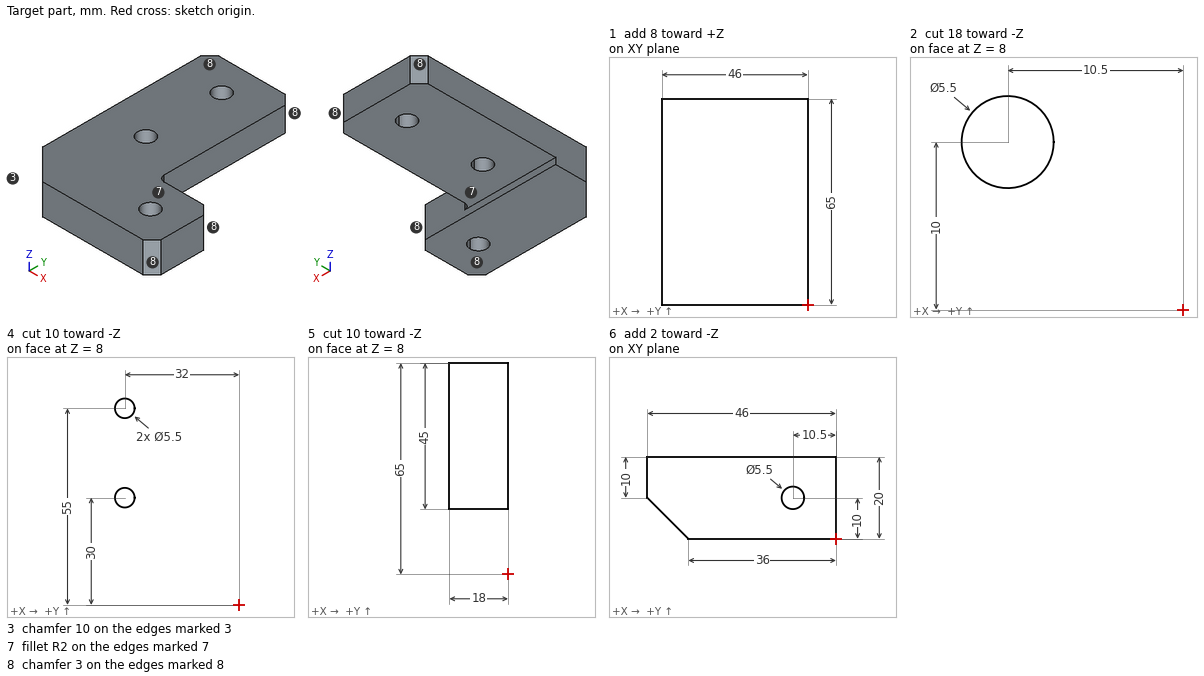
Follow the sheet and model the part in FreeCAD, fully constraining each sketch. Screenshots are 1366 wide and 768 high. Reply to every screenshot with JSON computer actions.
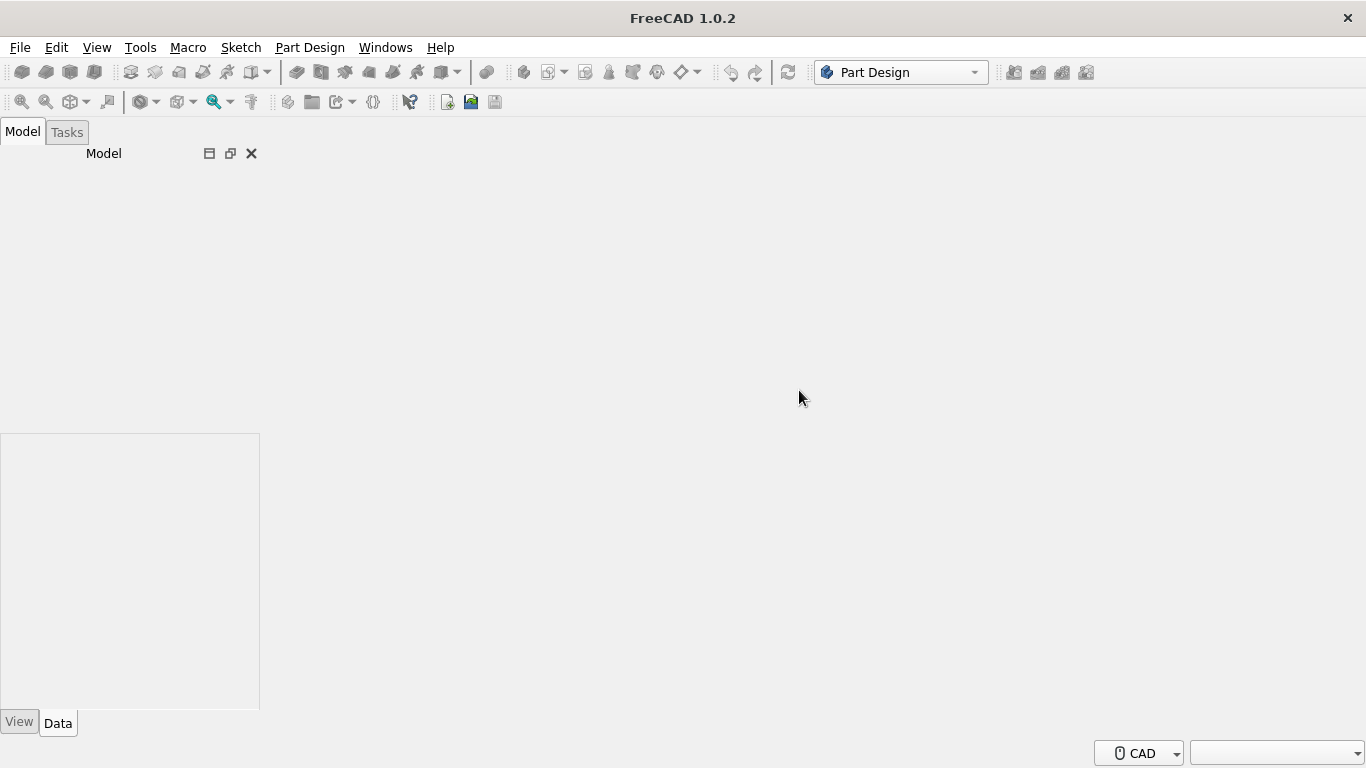
{"action": "left_click", "coordinate": [448, 102]}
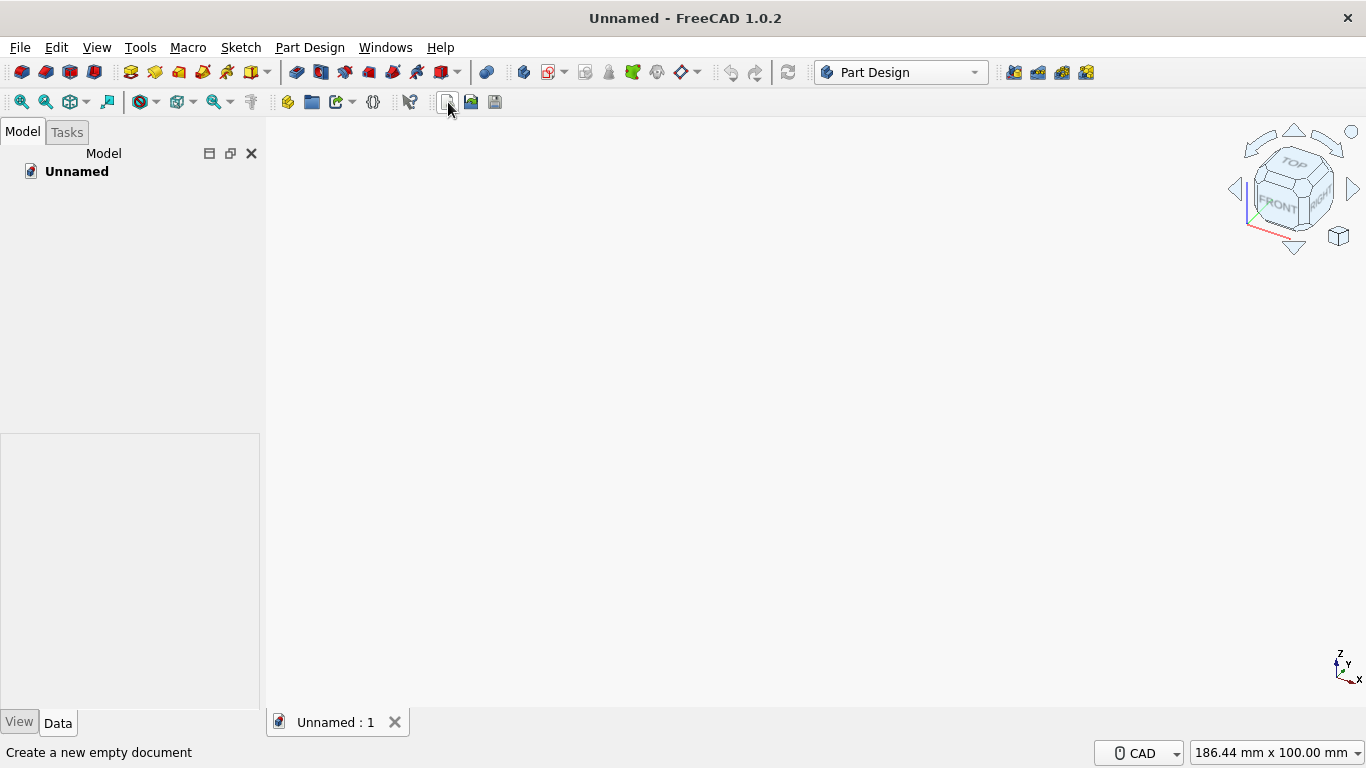
{"action": "left_click", "coordinate": [548, 72]}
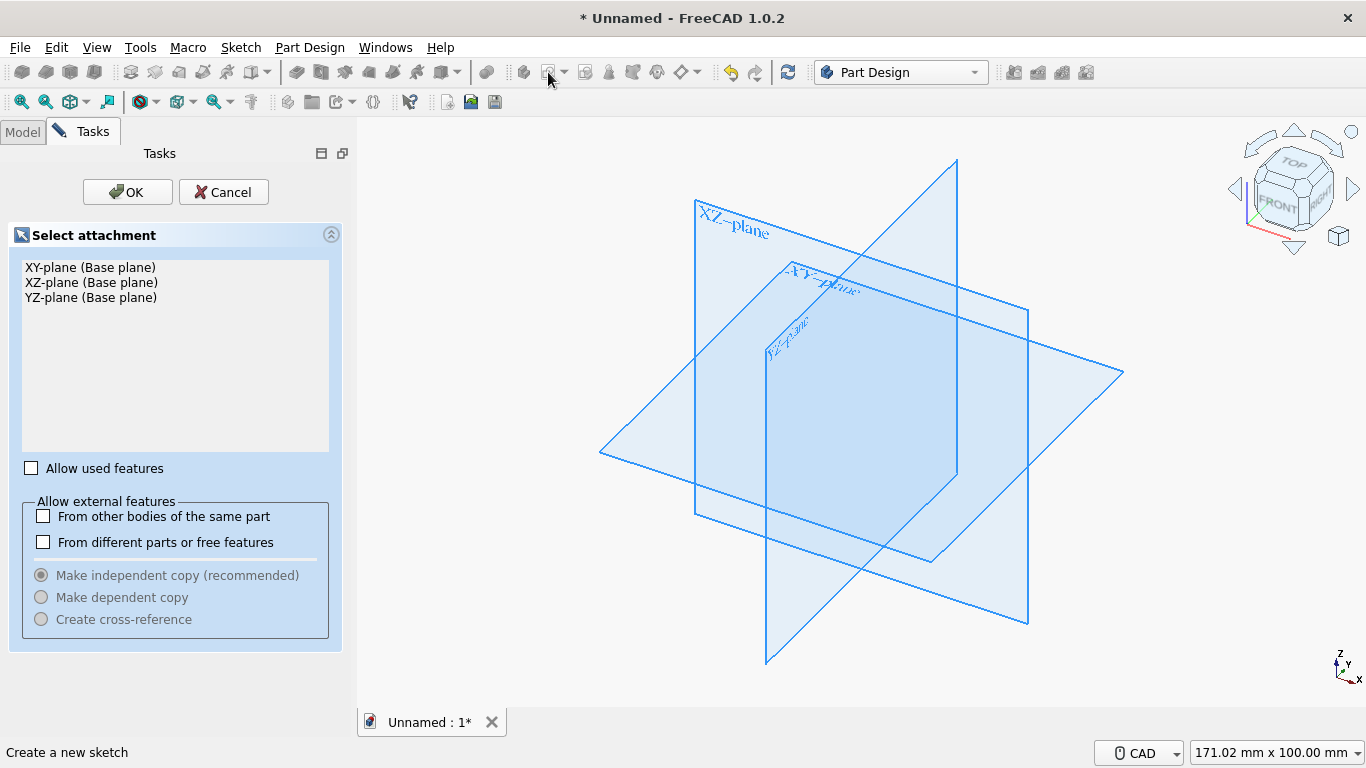
{"action": "left_click", "coordinate": [82, 268]}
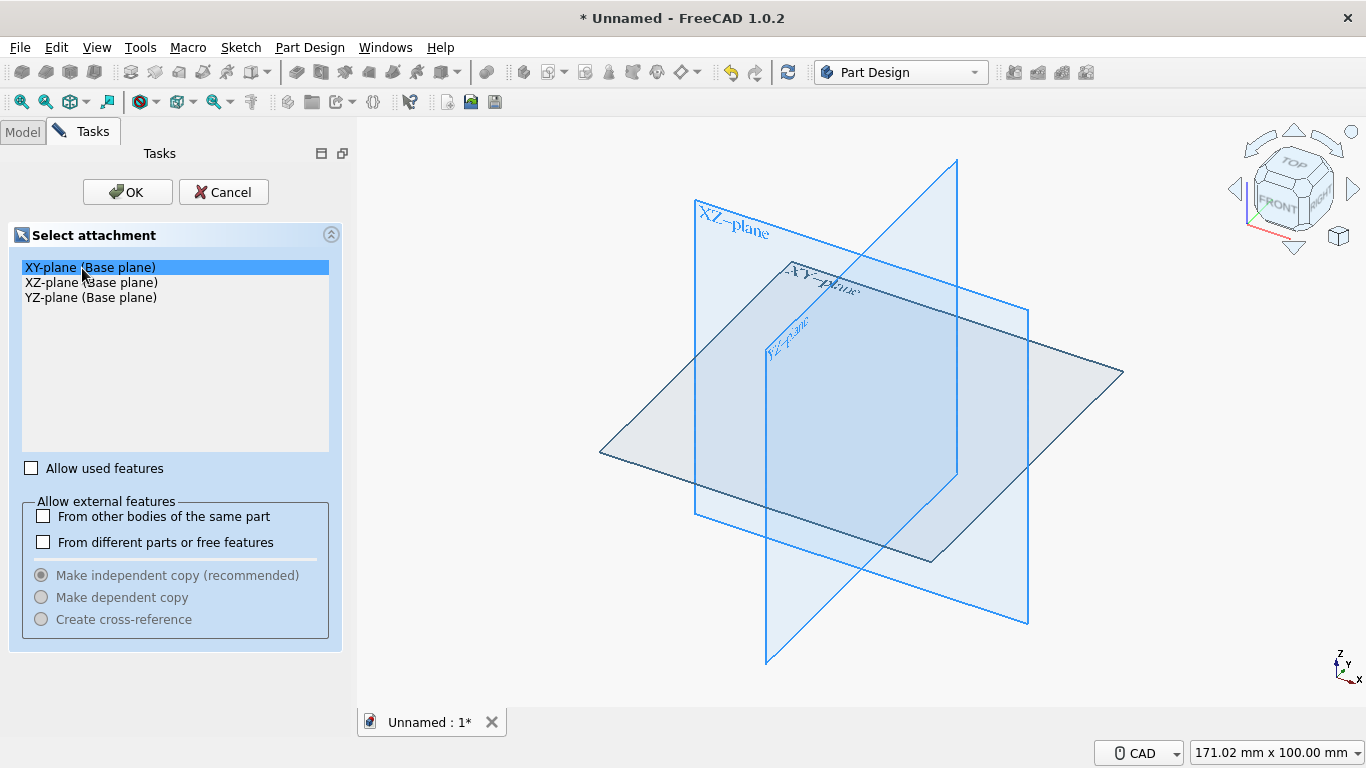
{"action": "left_click", "coordinate": [128, 192]}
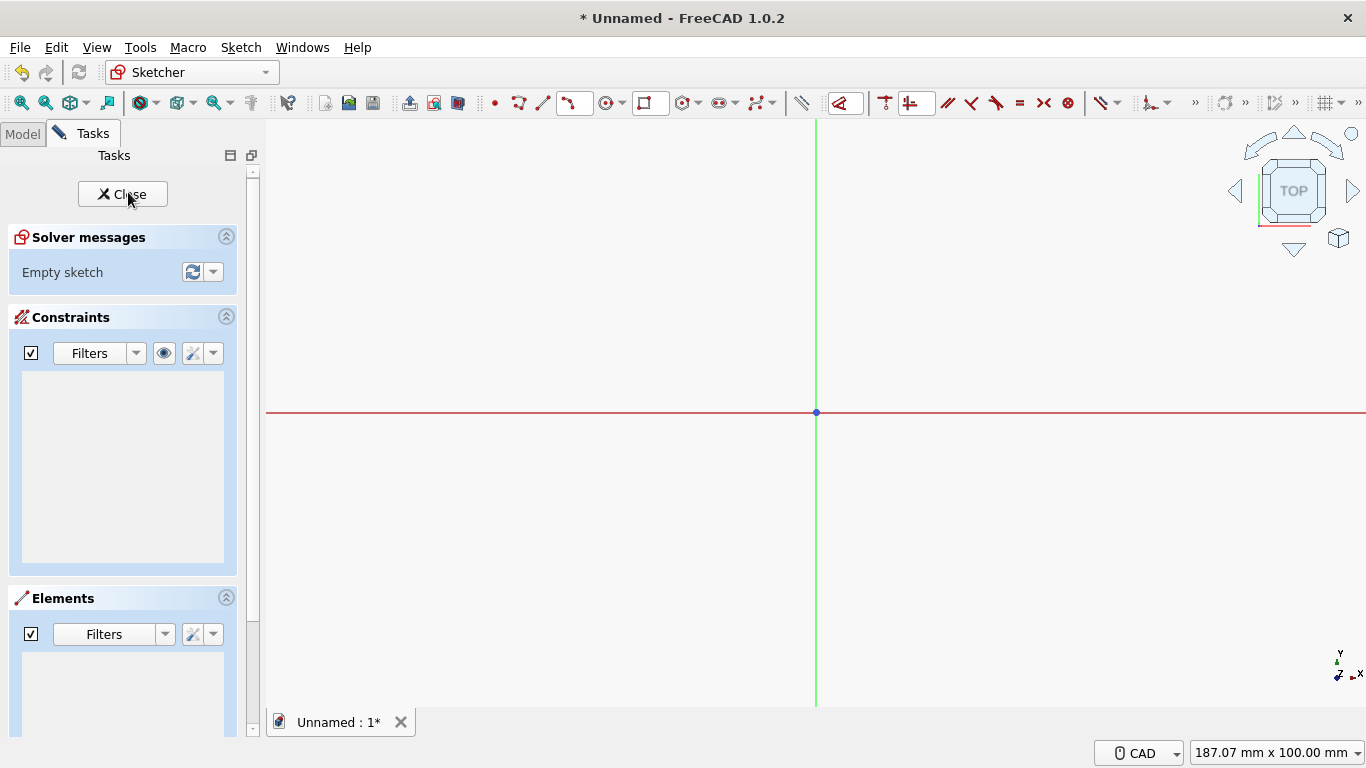
{"action": "scroll", "coordinate": [883, 679], "scroll_direction": "down", "scroll_amount": 2}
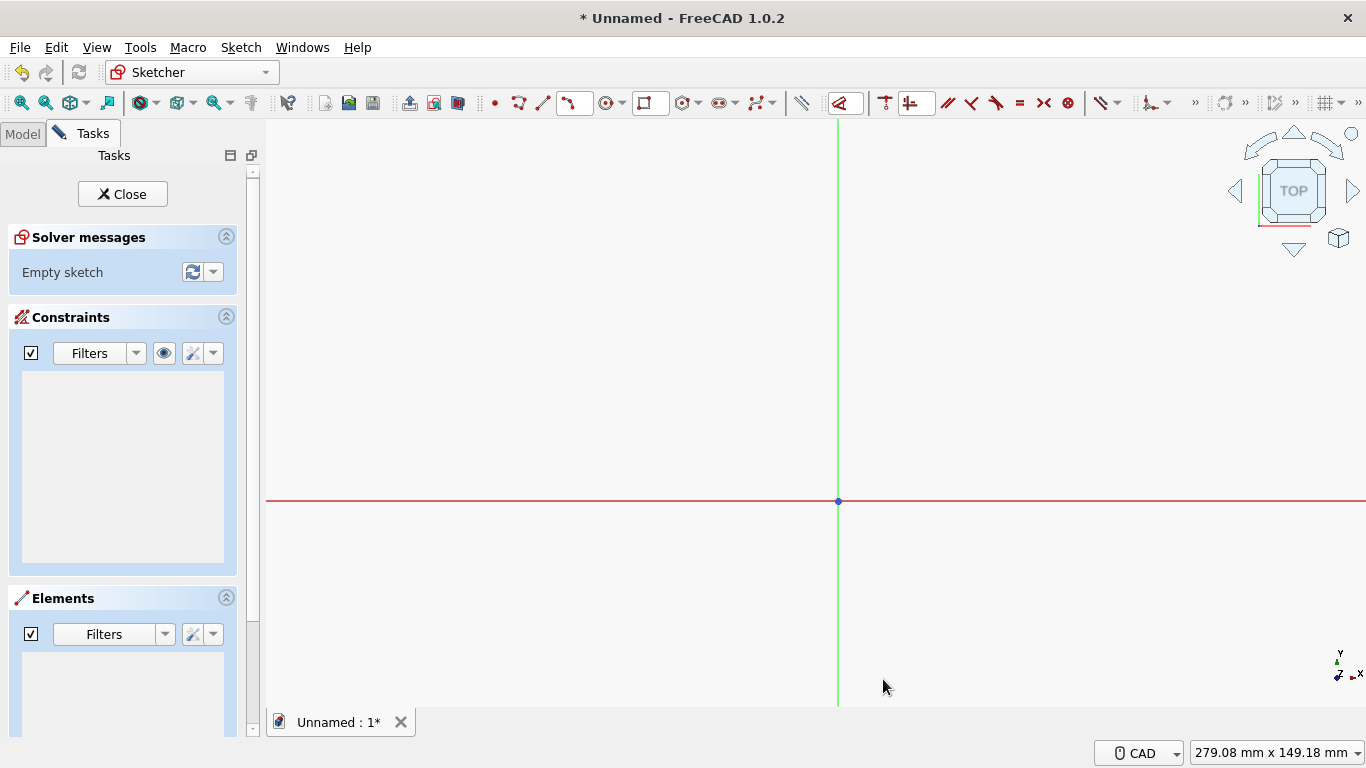
{"action": "scroll", "coordinate": [748, 291], "scroll_direction": "up", "scroll_amount": 2}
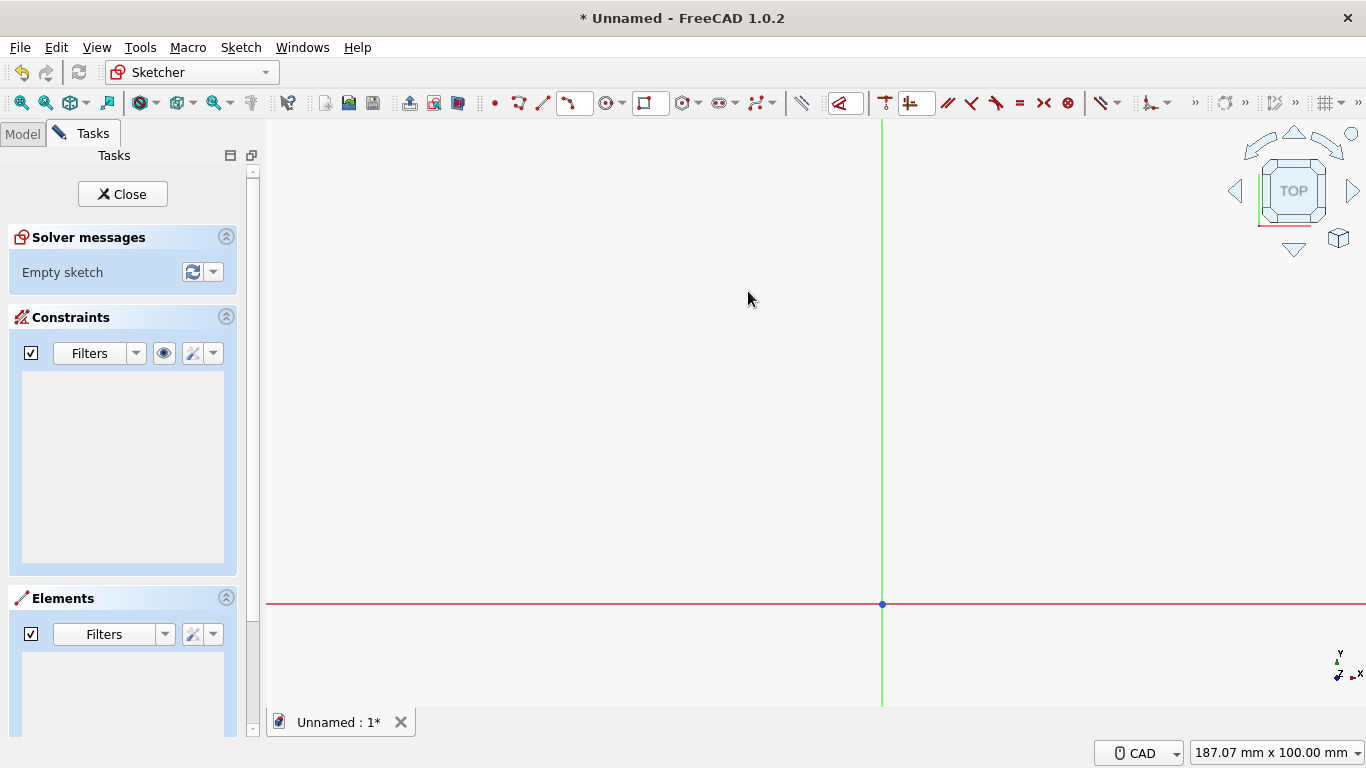
{"action": "key", "text": "g r"}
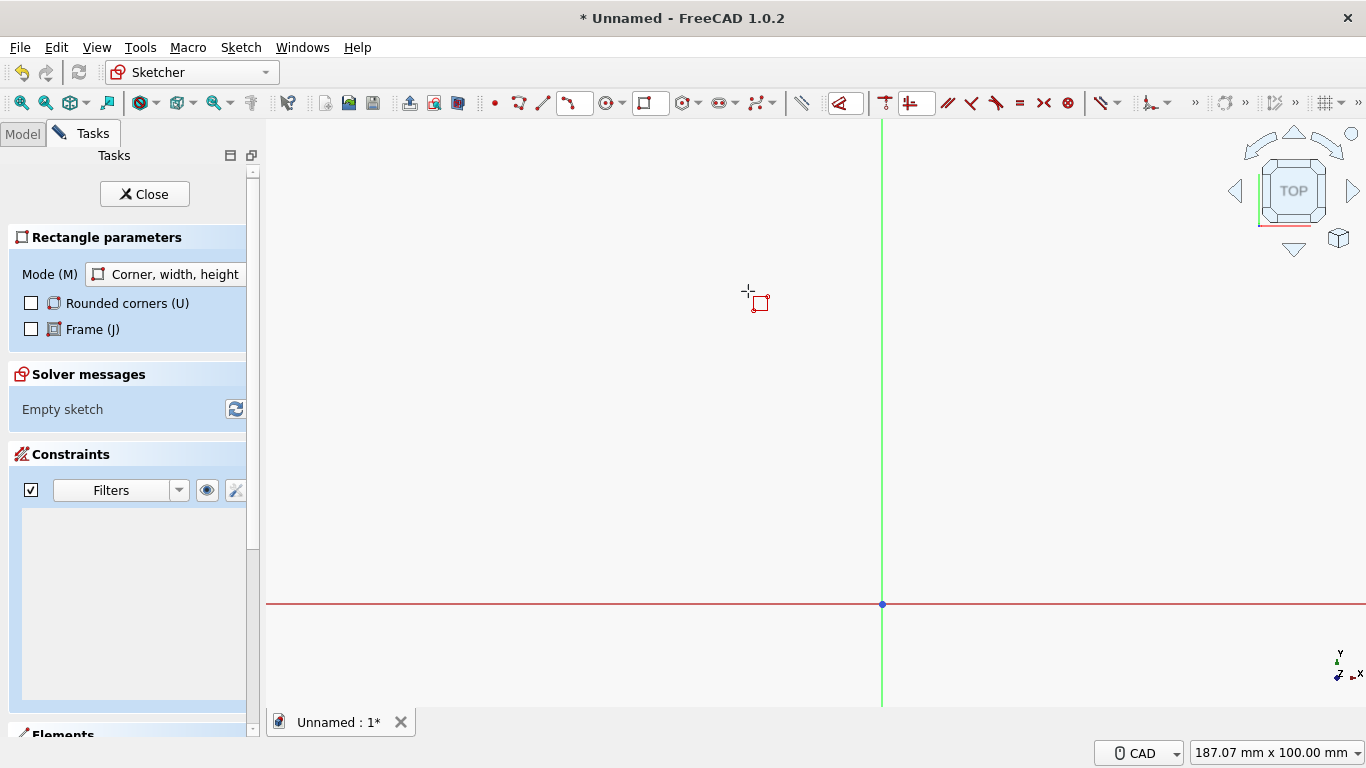
{"action": "left_click", "coordinate": [882, 604]}
{"action": "left_click", "coordinate": [612, 222]}
{"action": "key", "text": "Escape"}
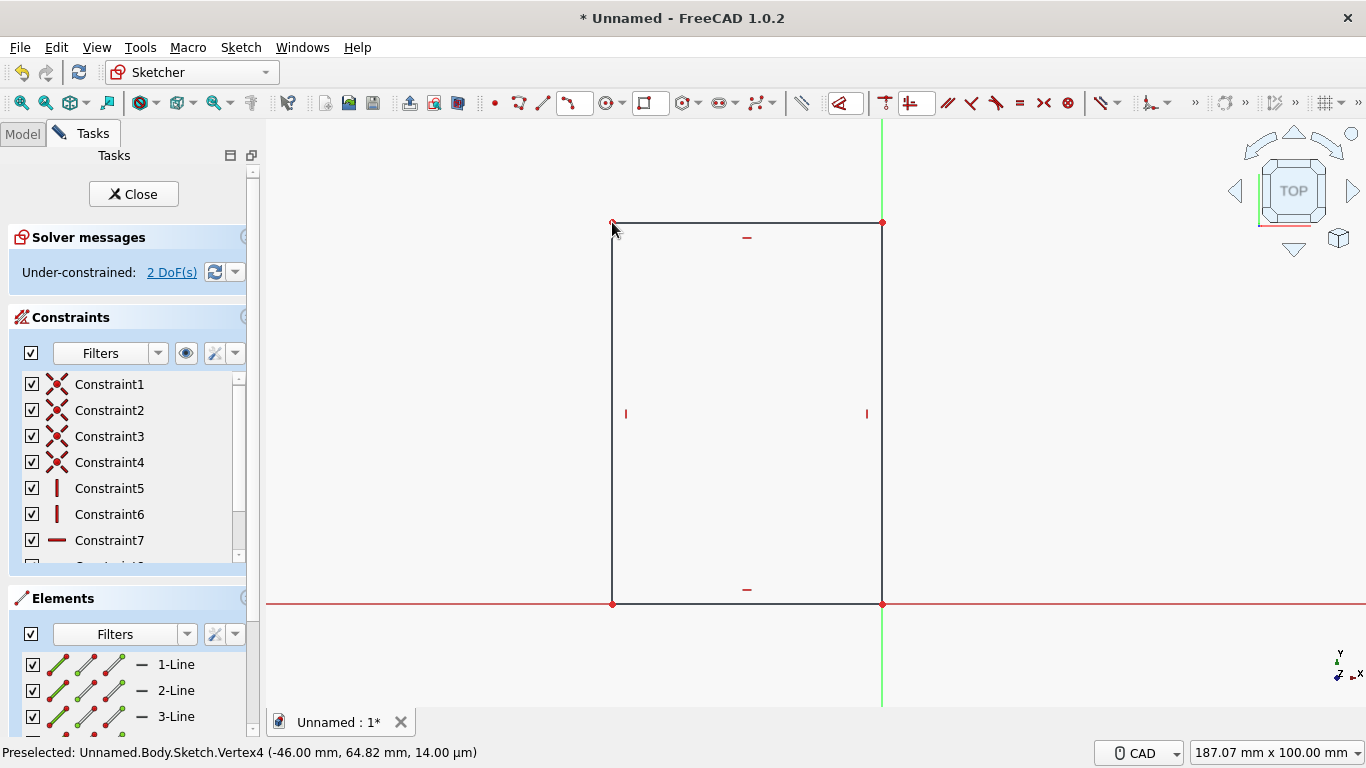
{"action": "left_click", "coordinate": [882, 490]}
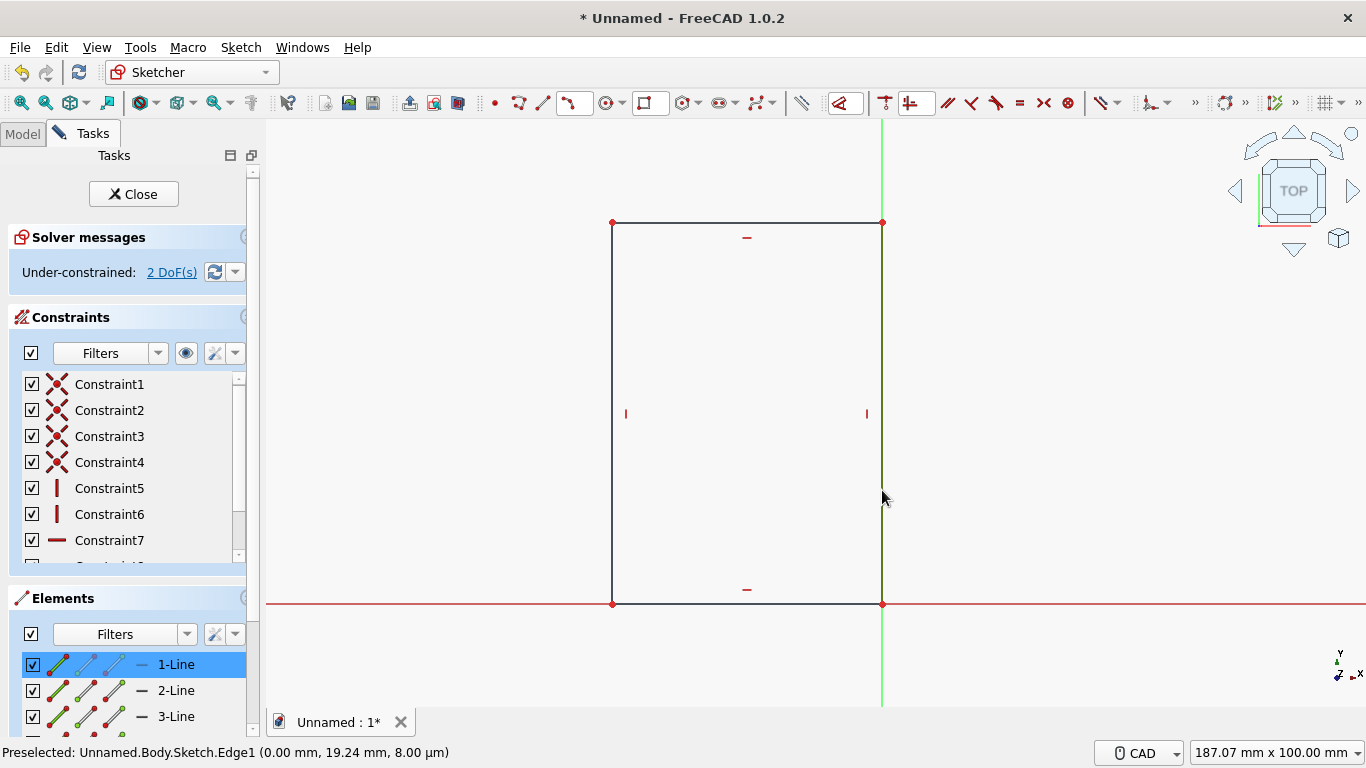
{"action": "key", "text": "i"}